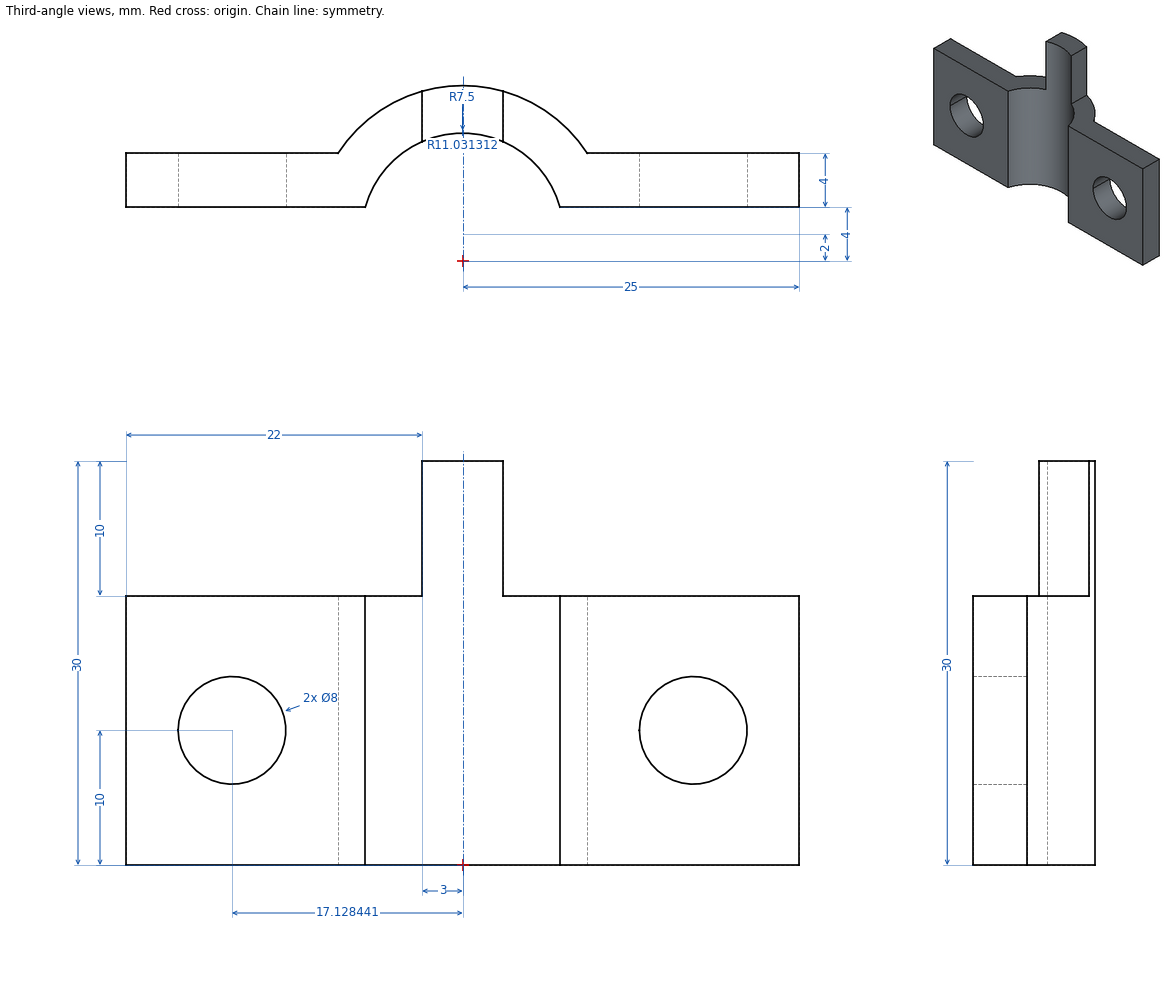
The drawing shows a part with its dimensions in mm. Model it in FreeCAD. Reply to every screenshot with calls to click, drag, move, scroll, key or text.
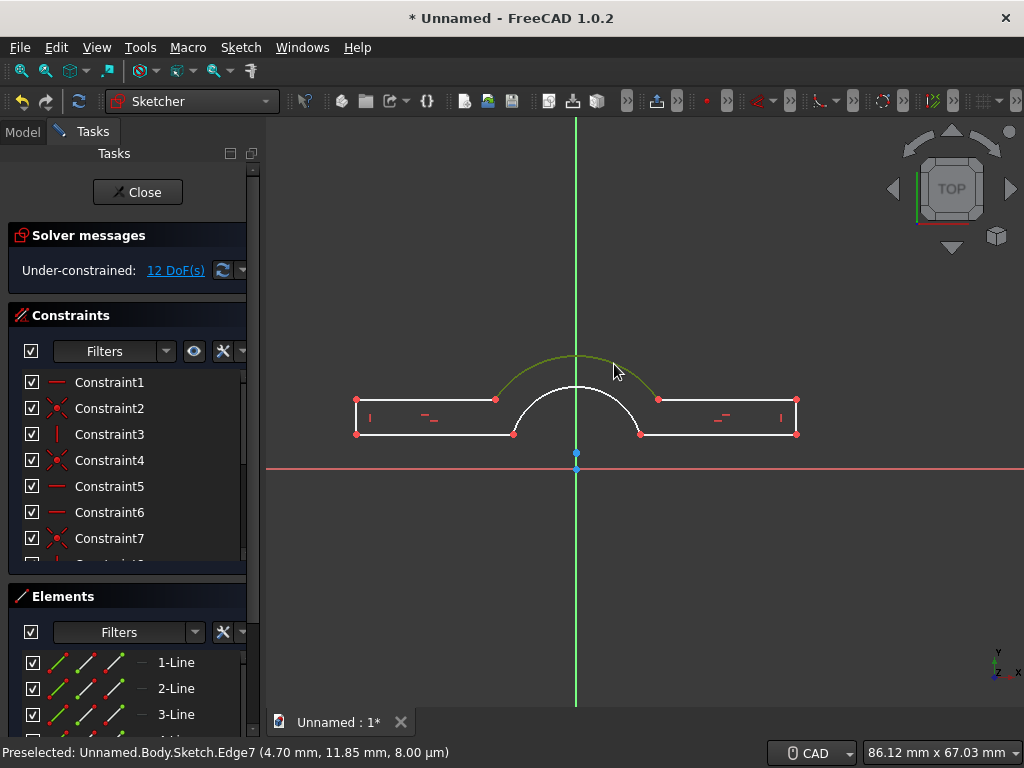
click(609, 396)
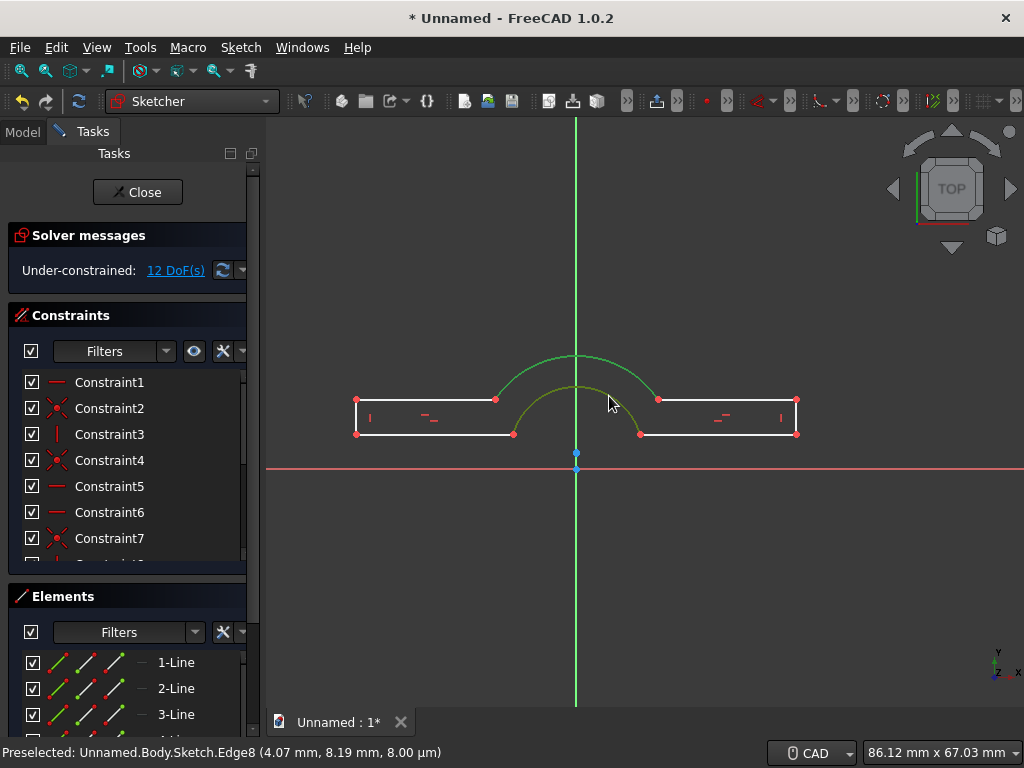
key(c)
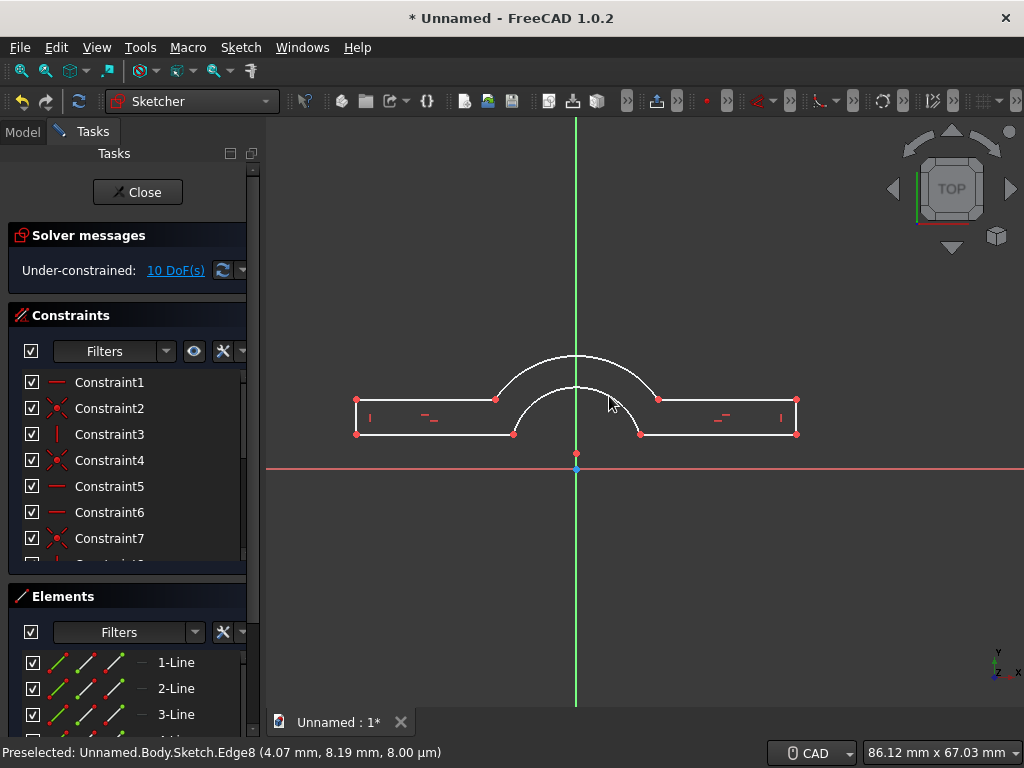
click(577, 454)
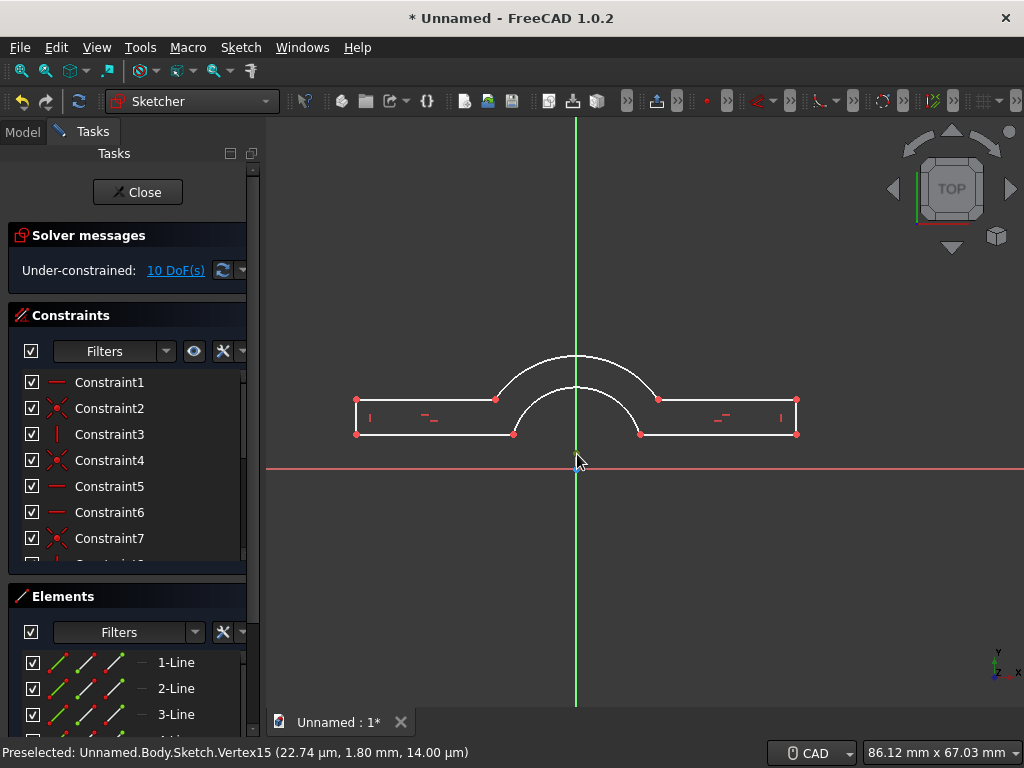
click(576, 641)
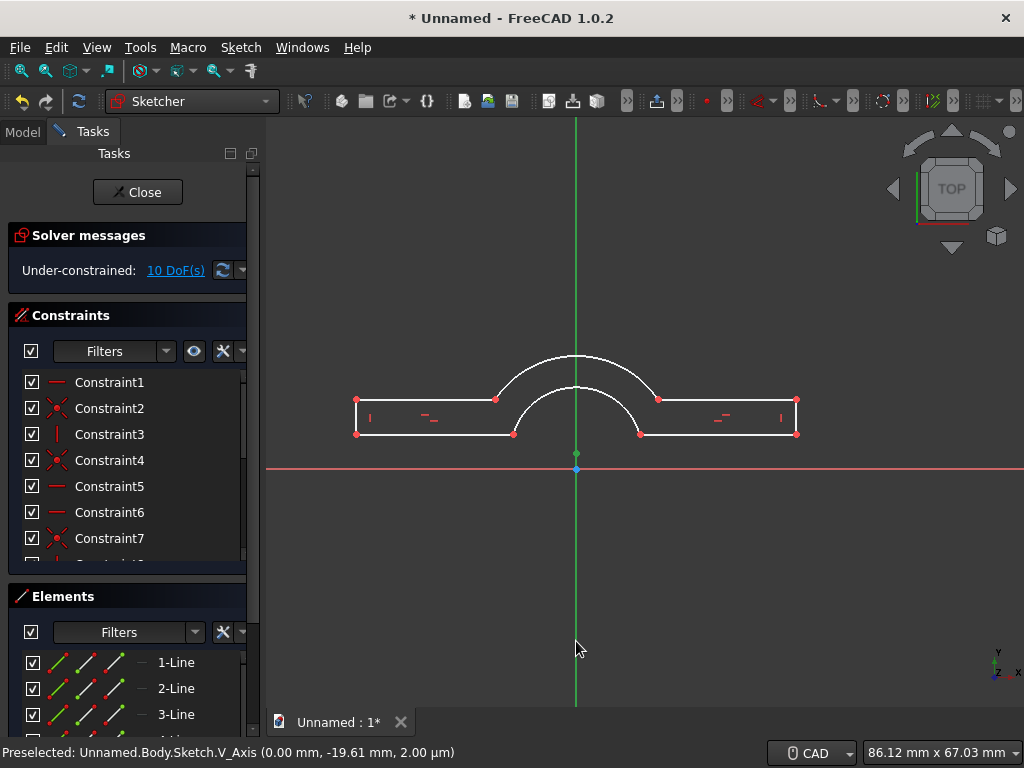
key(c)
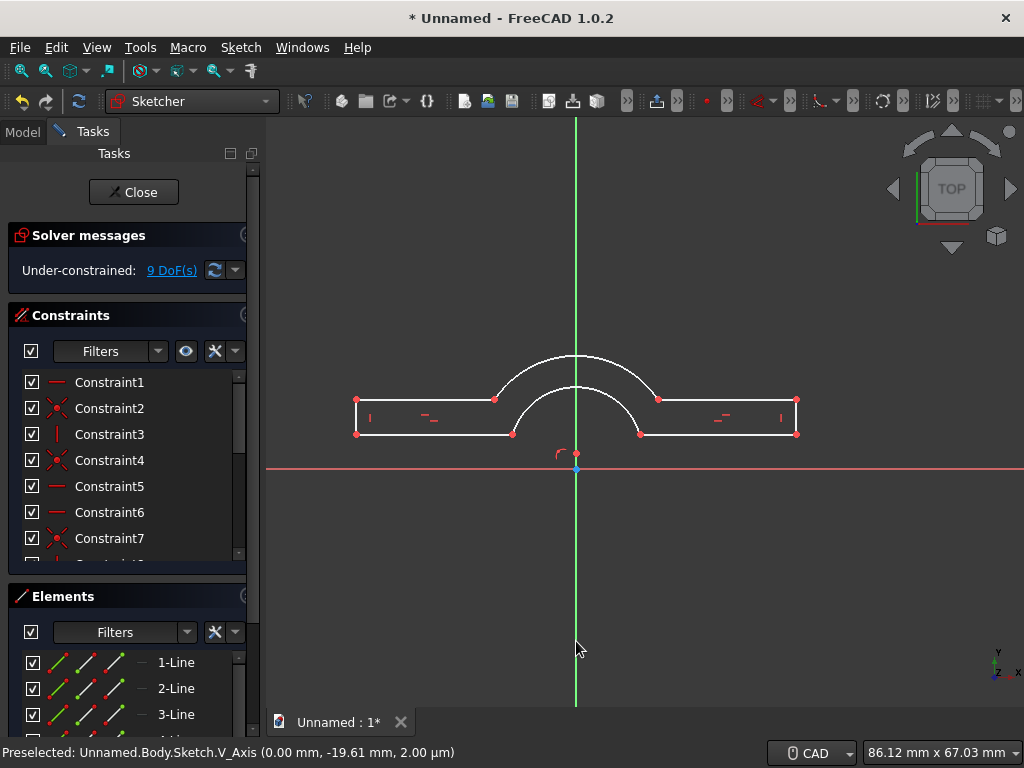
click(796, 400)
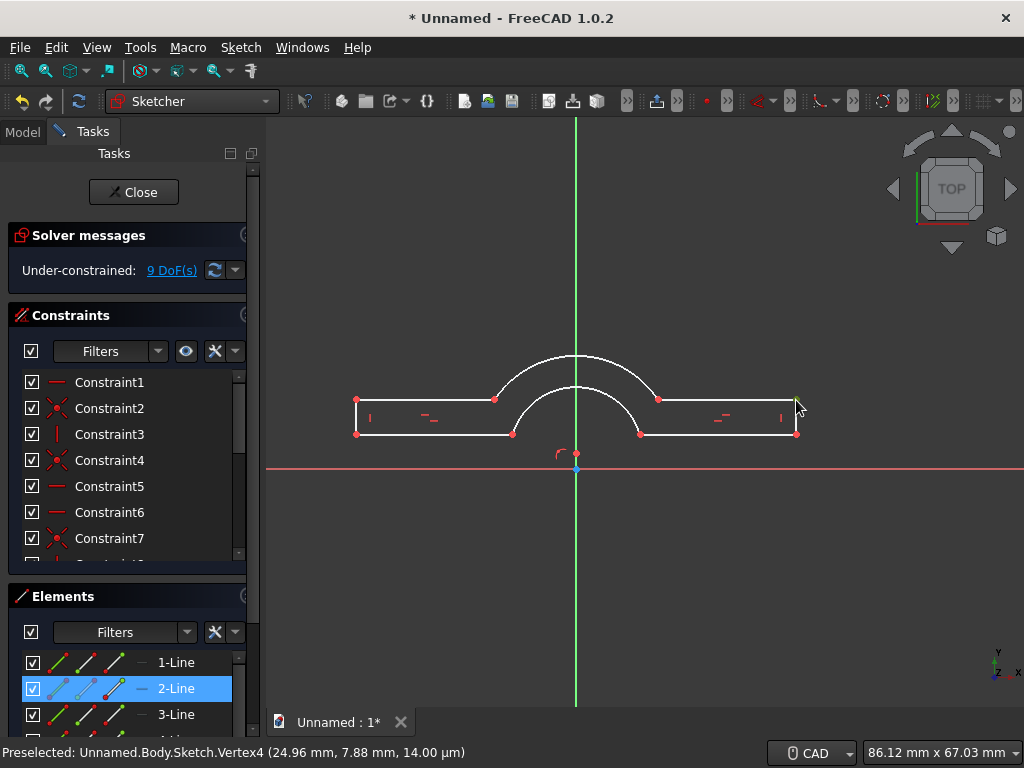
click(356, 400)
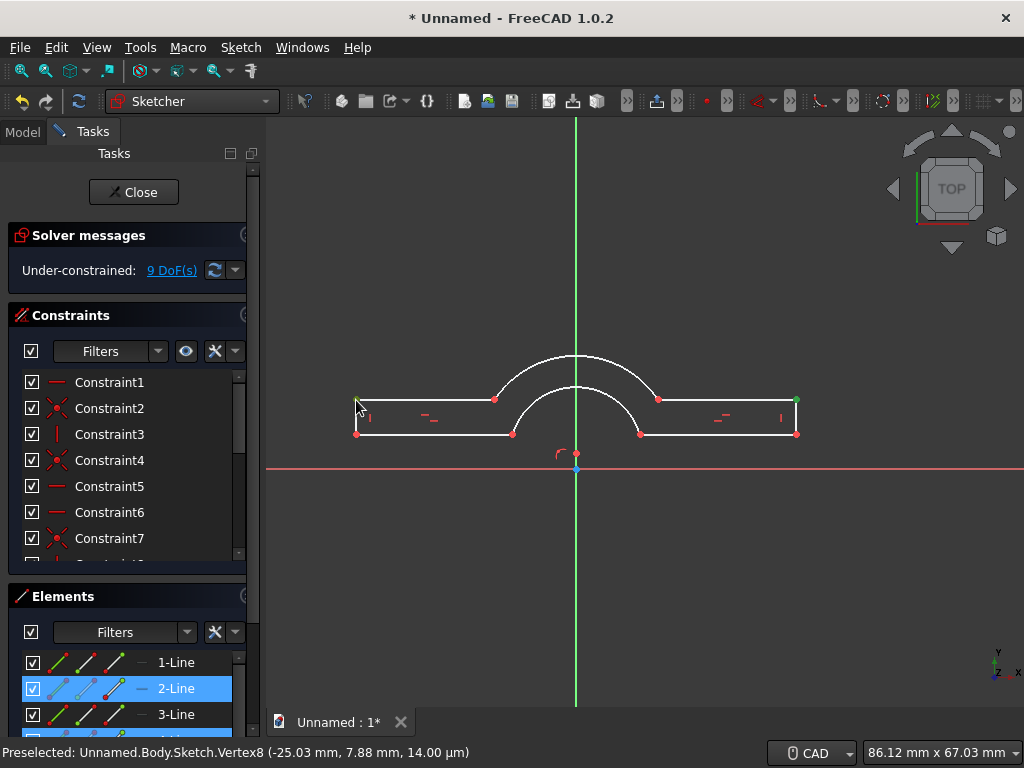
click(576, 641)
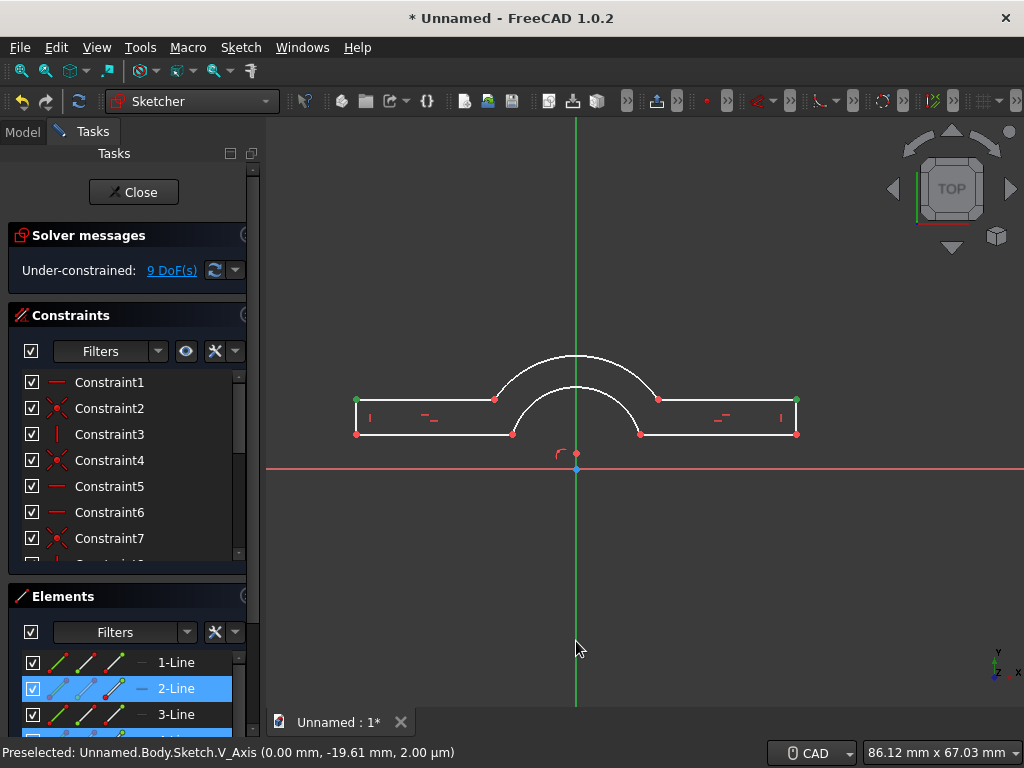
key(s)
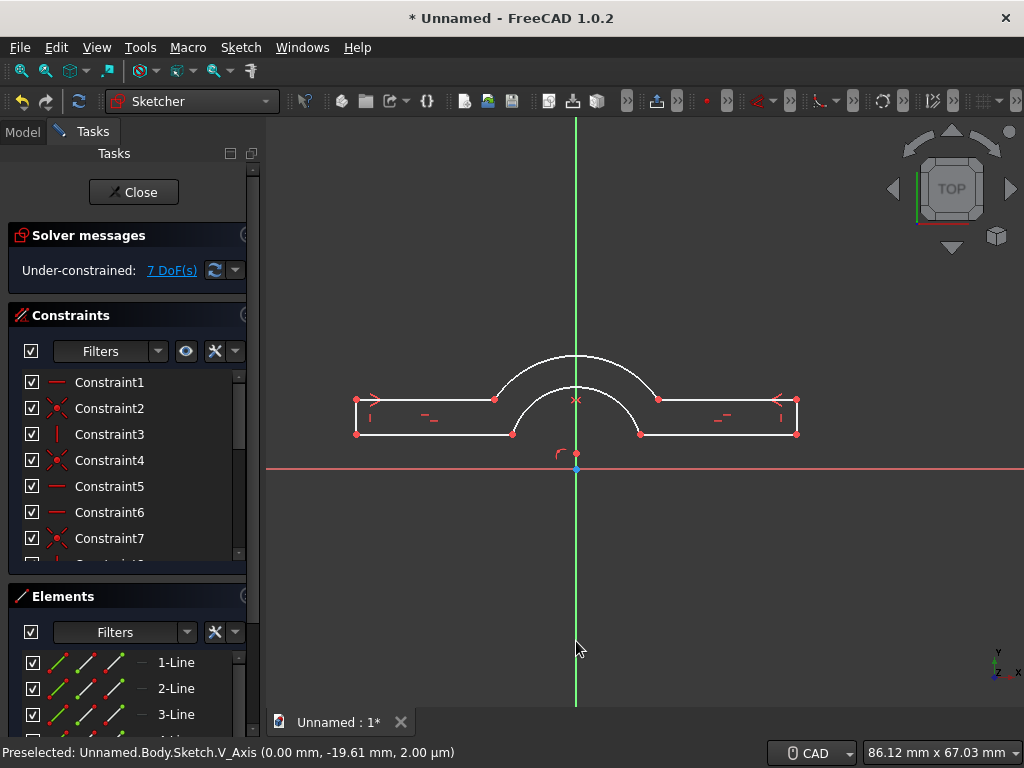
click(758, 102)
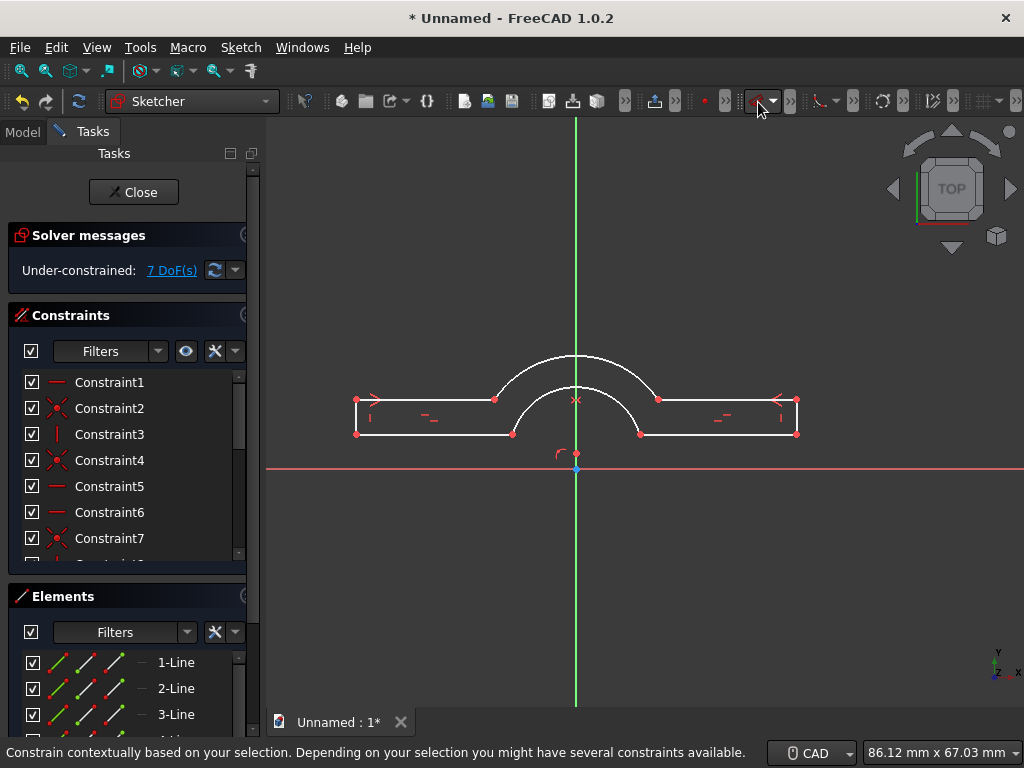
click(614, 363)
click(626, 333)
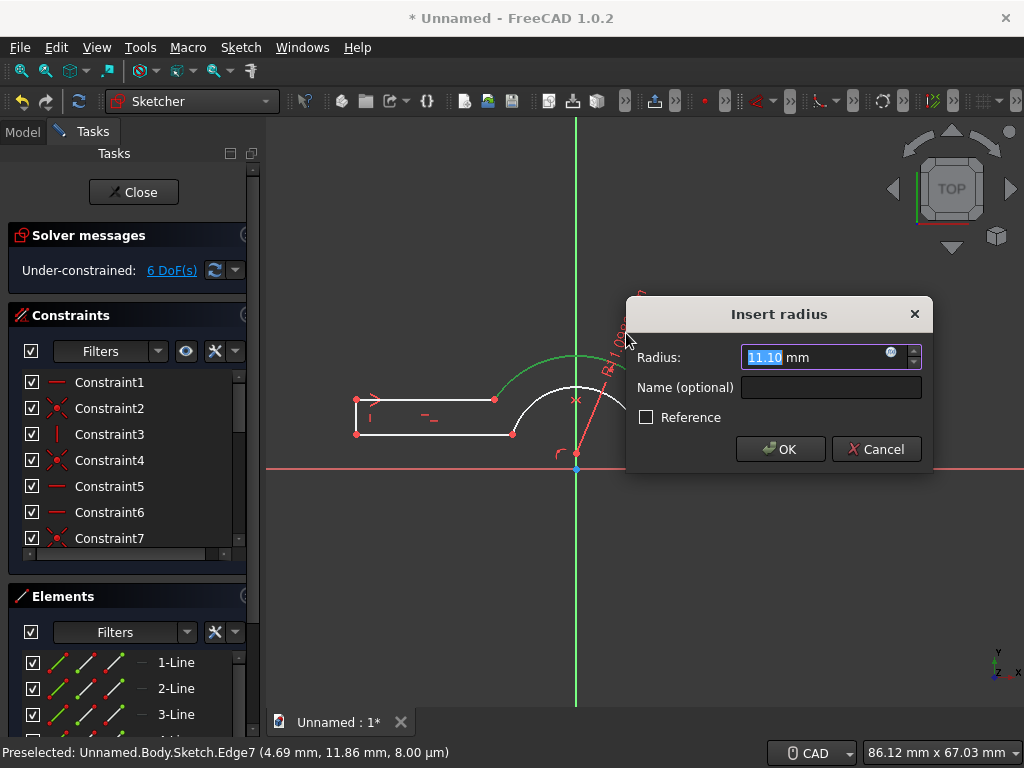
text(11.031312)
key(Return)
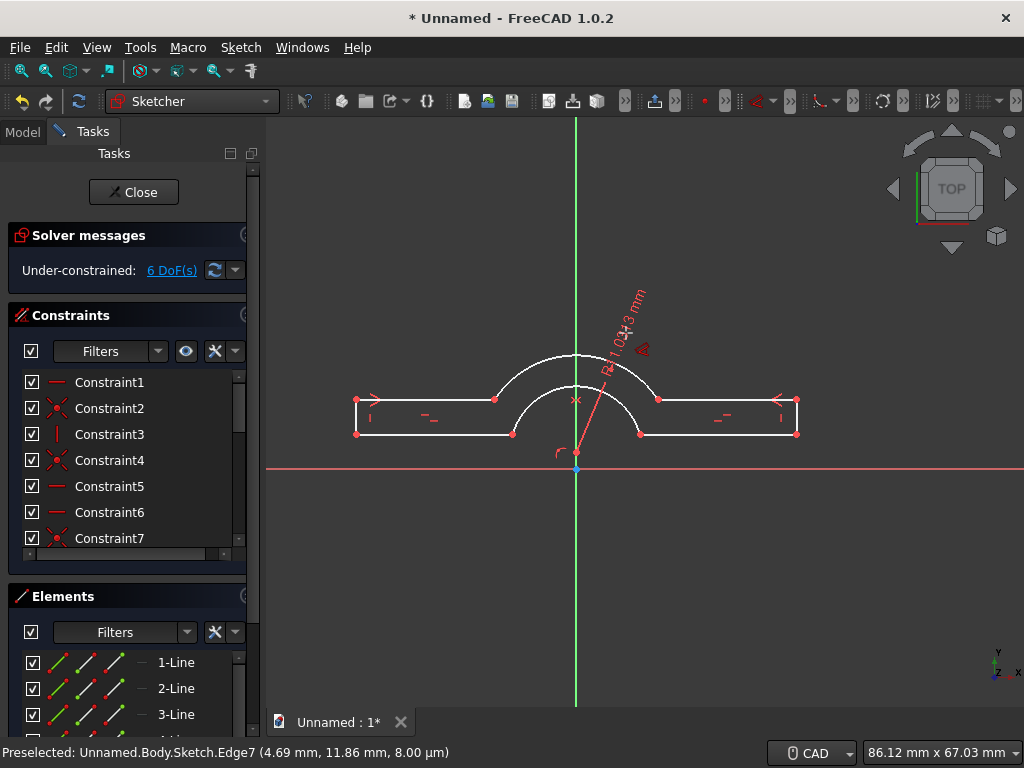
click(609, 395)
click(662, 501)